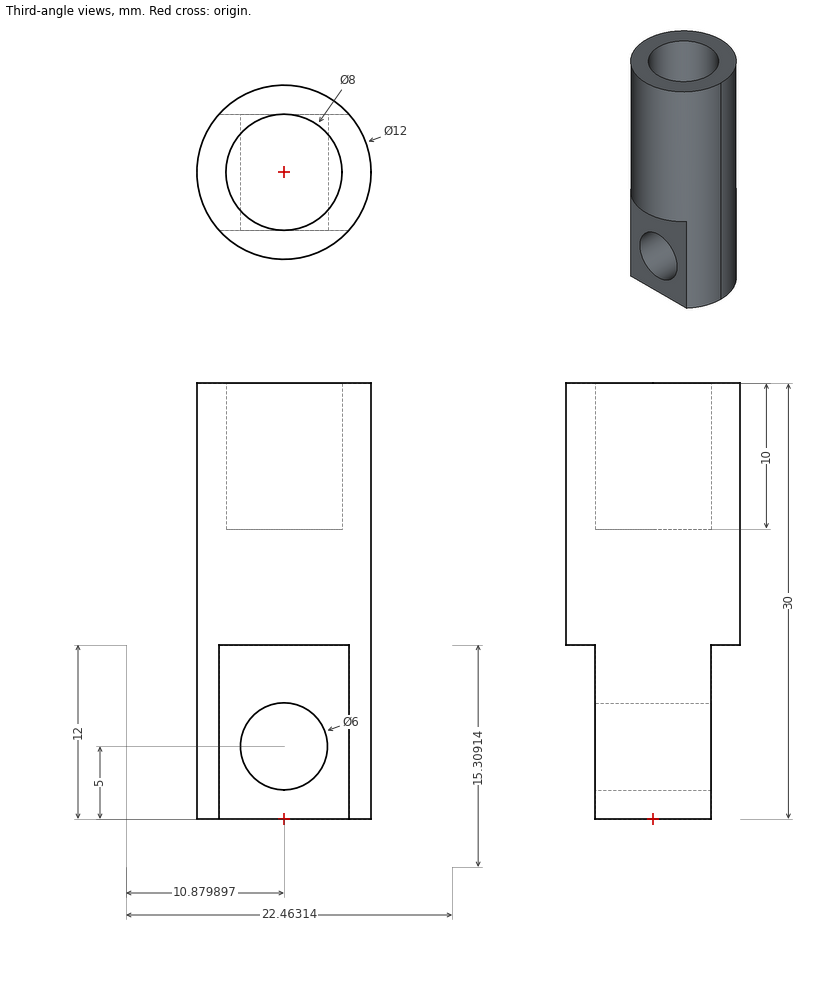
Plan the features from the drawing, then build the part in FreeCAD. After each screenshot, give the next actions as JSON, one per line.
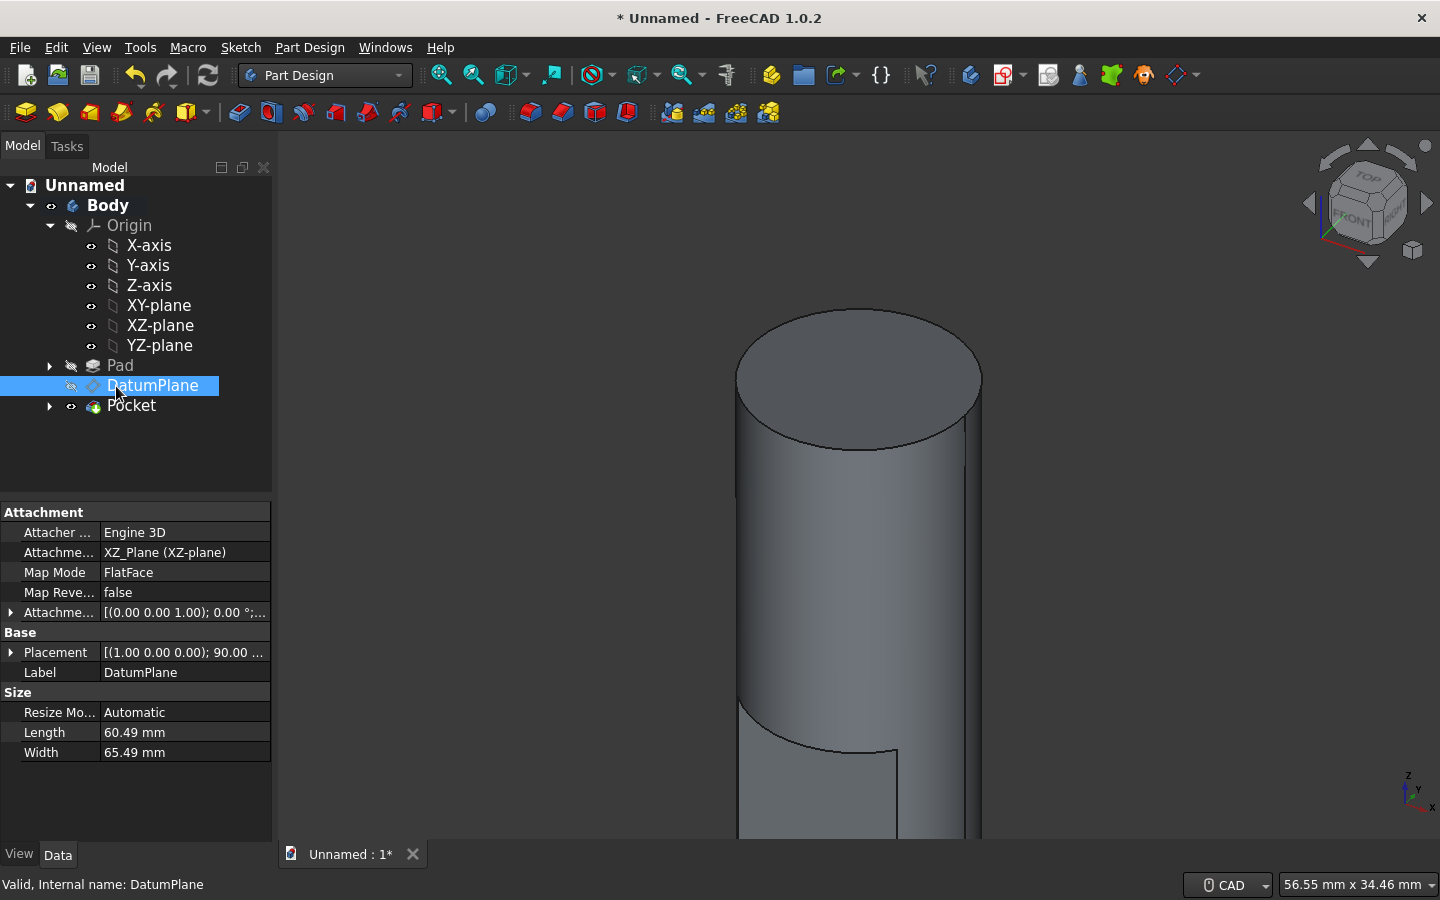
{"action": "left_click", "coordinate": [442, 76]}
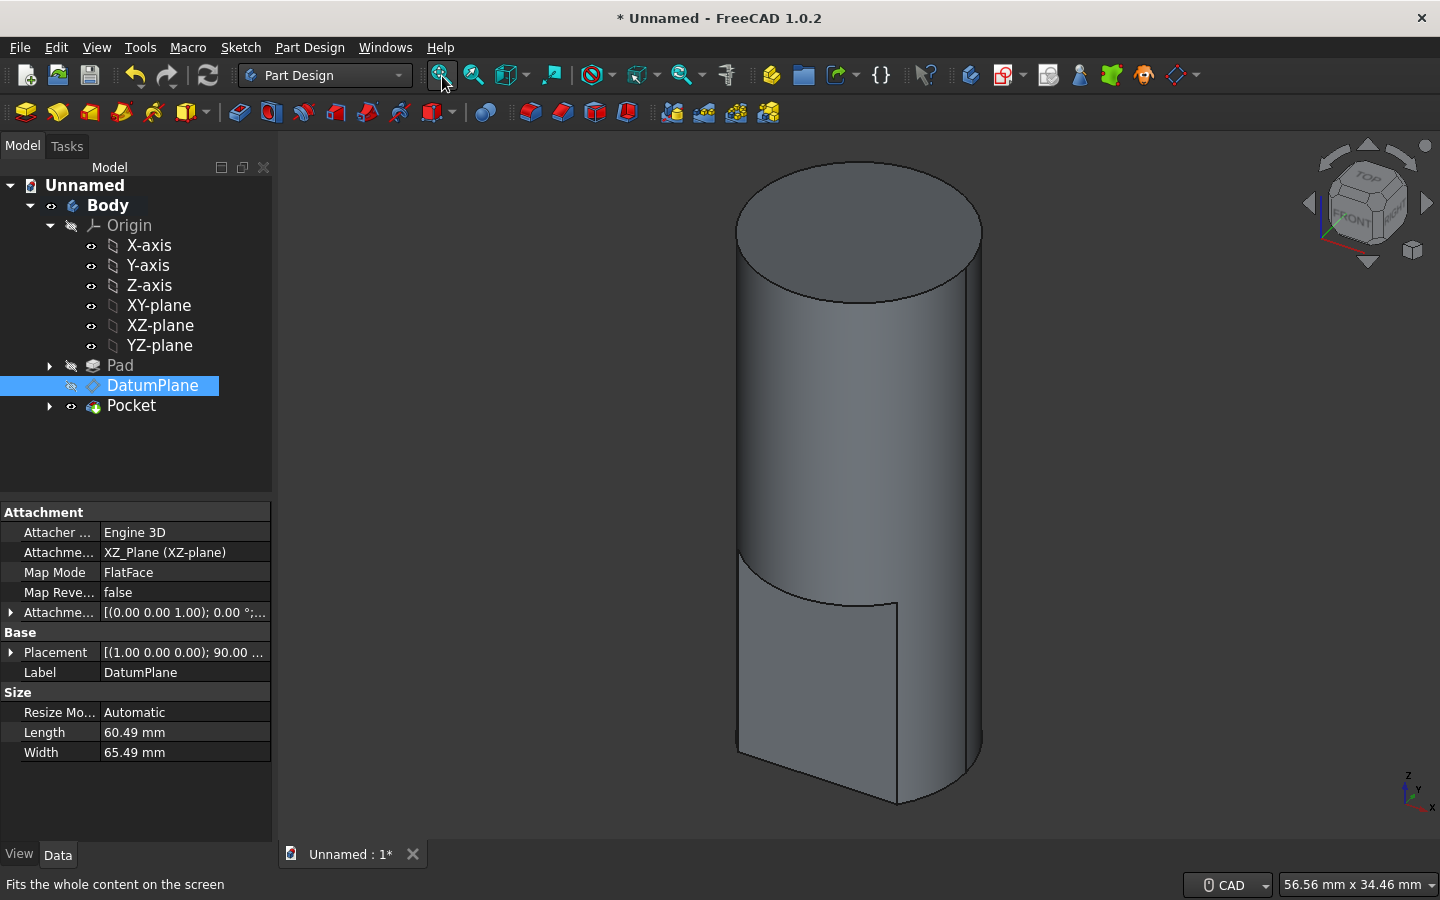
{"action": "left_click", "coordinate": [116, 406]}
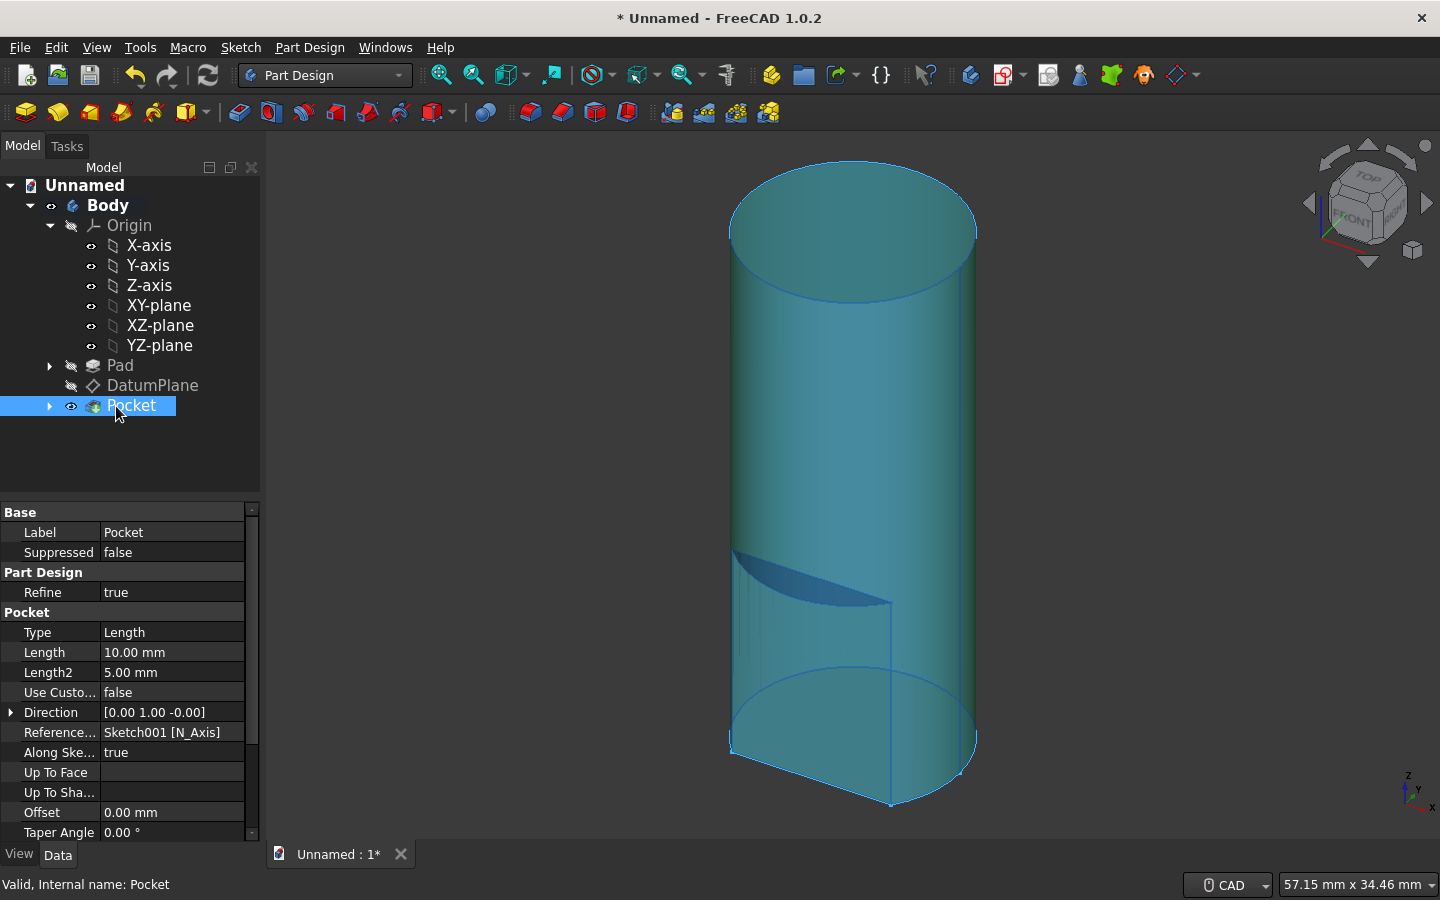
{"action": "left_click", "coordinate": [672, 112]}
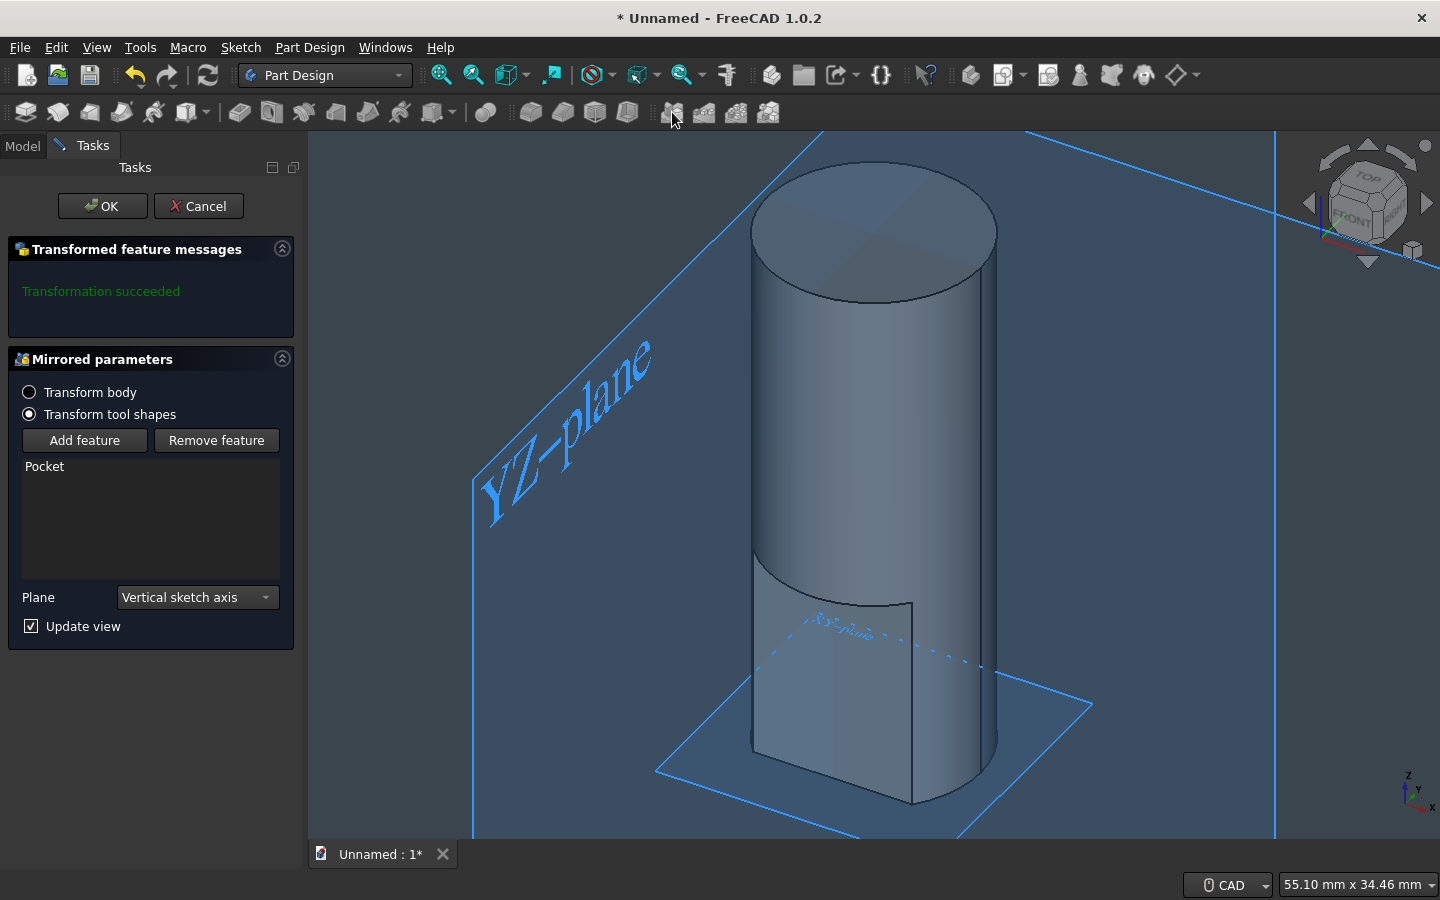
{"action": "left_click", "coordinate": [198, 598]}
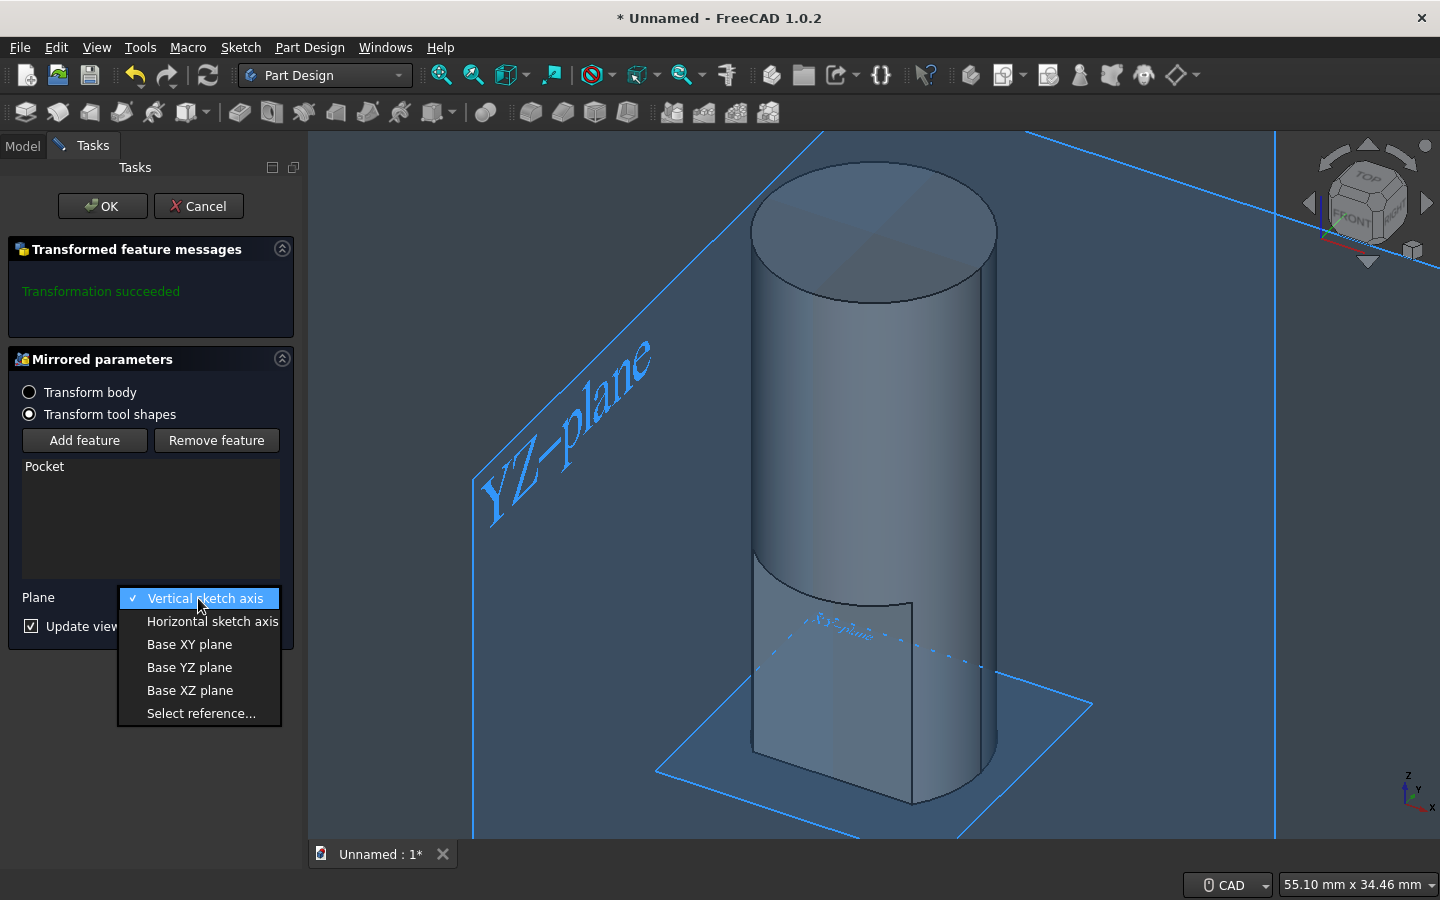
{"action": "left_click", "coordinate": [198, 690]}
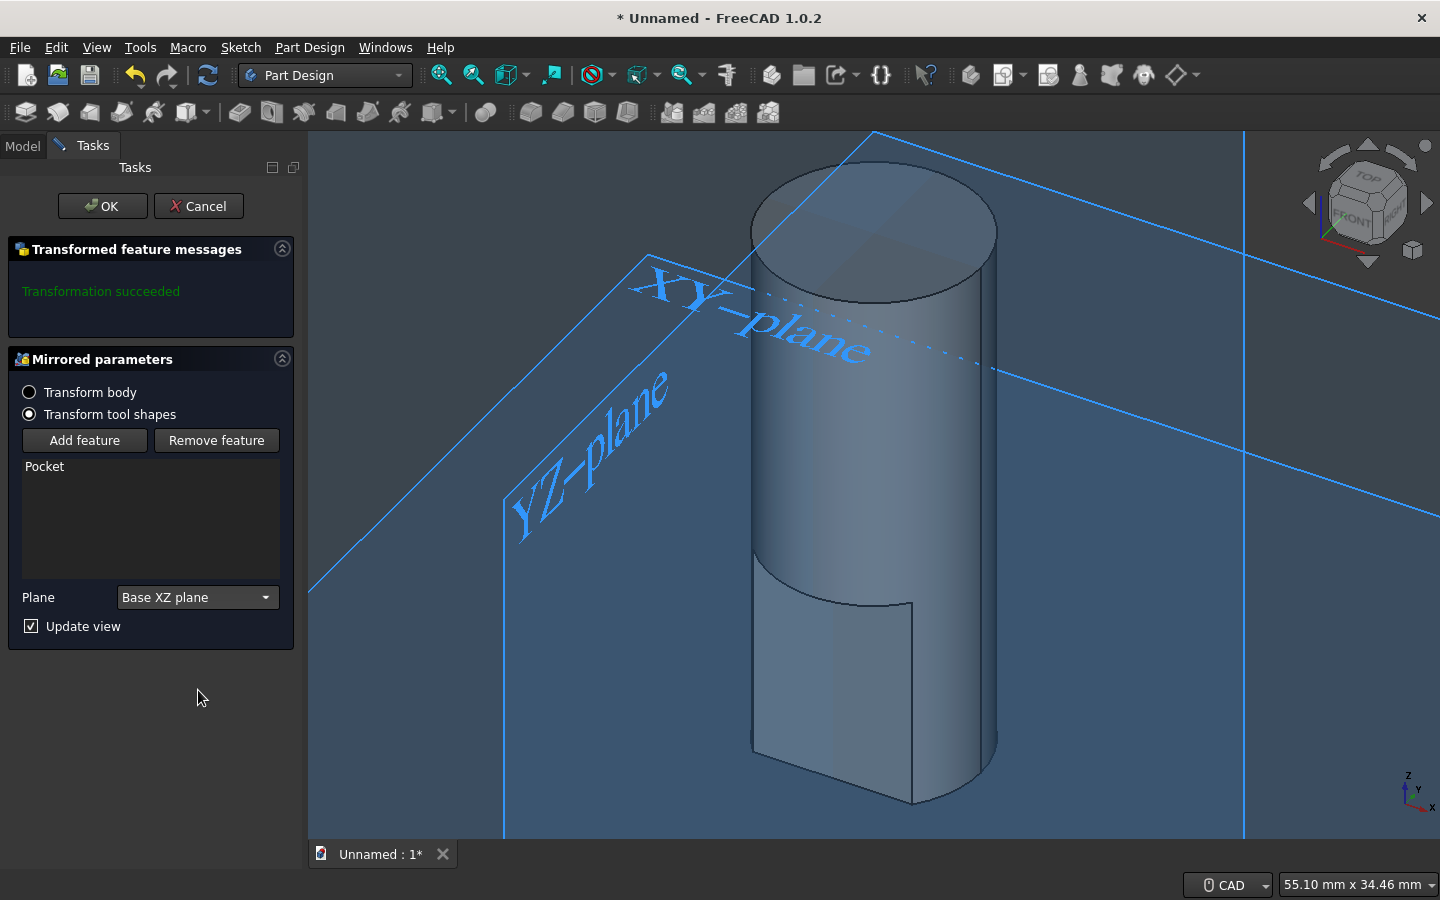
{"action": "left_click", "coordinate": [103, 206]}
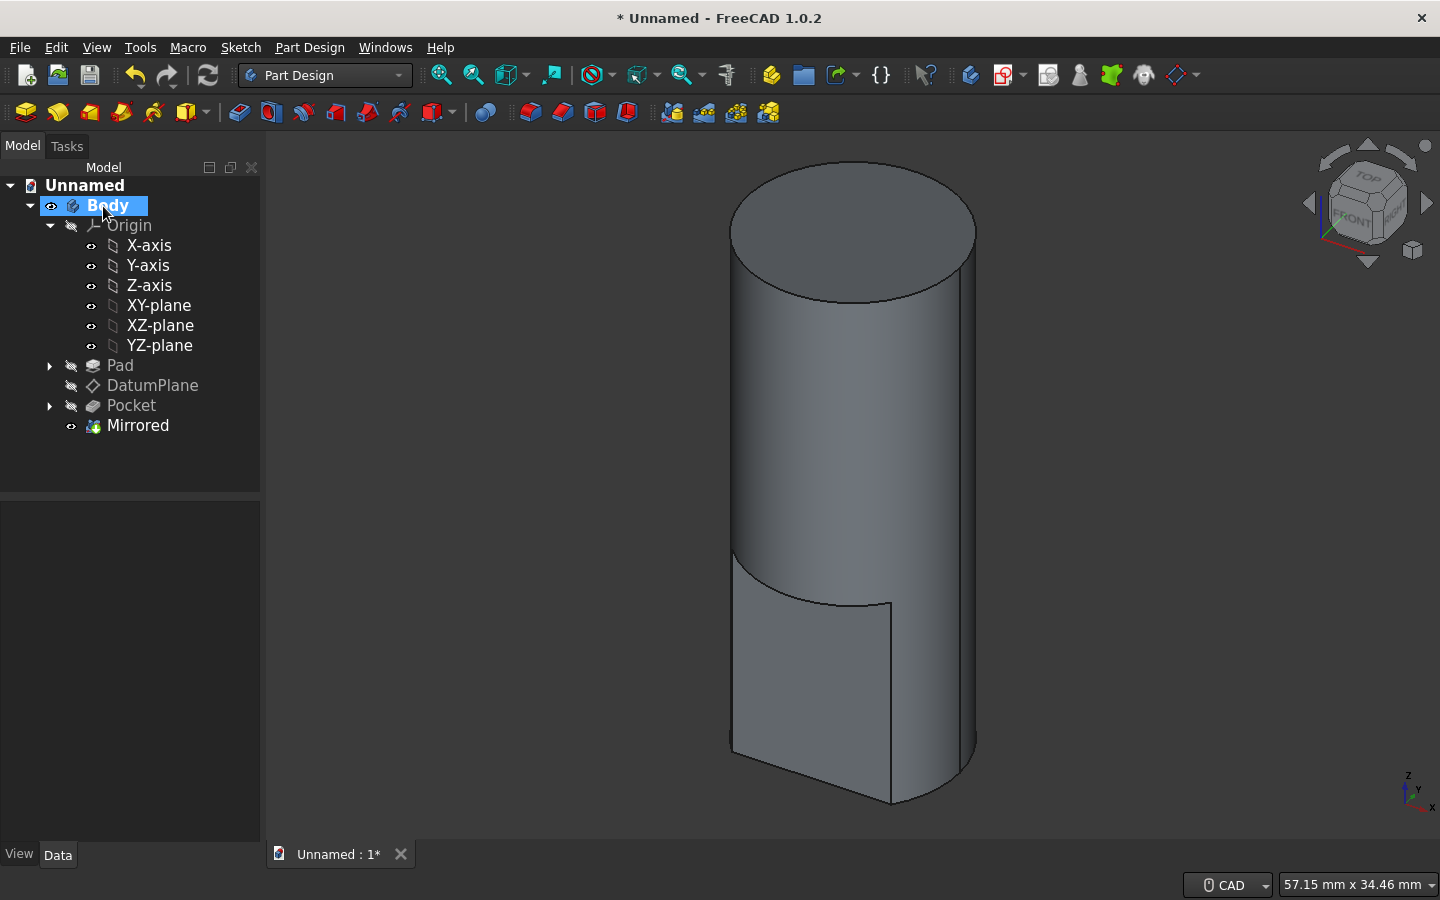
{"action": "left_click", "coordinate": [812, 676]}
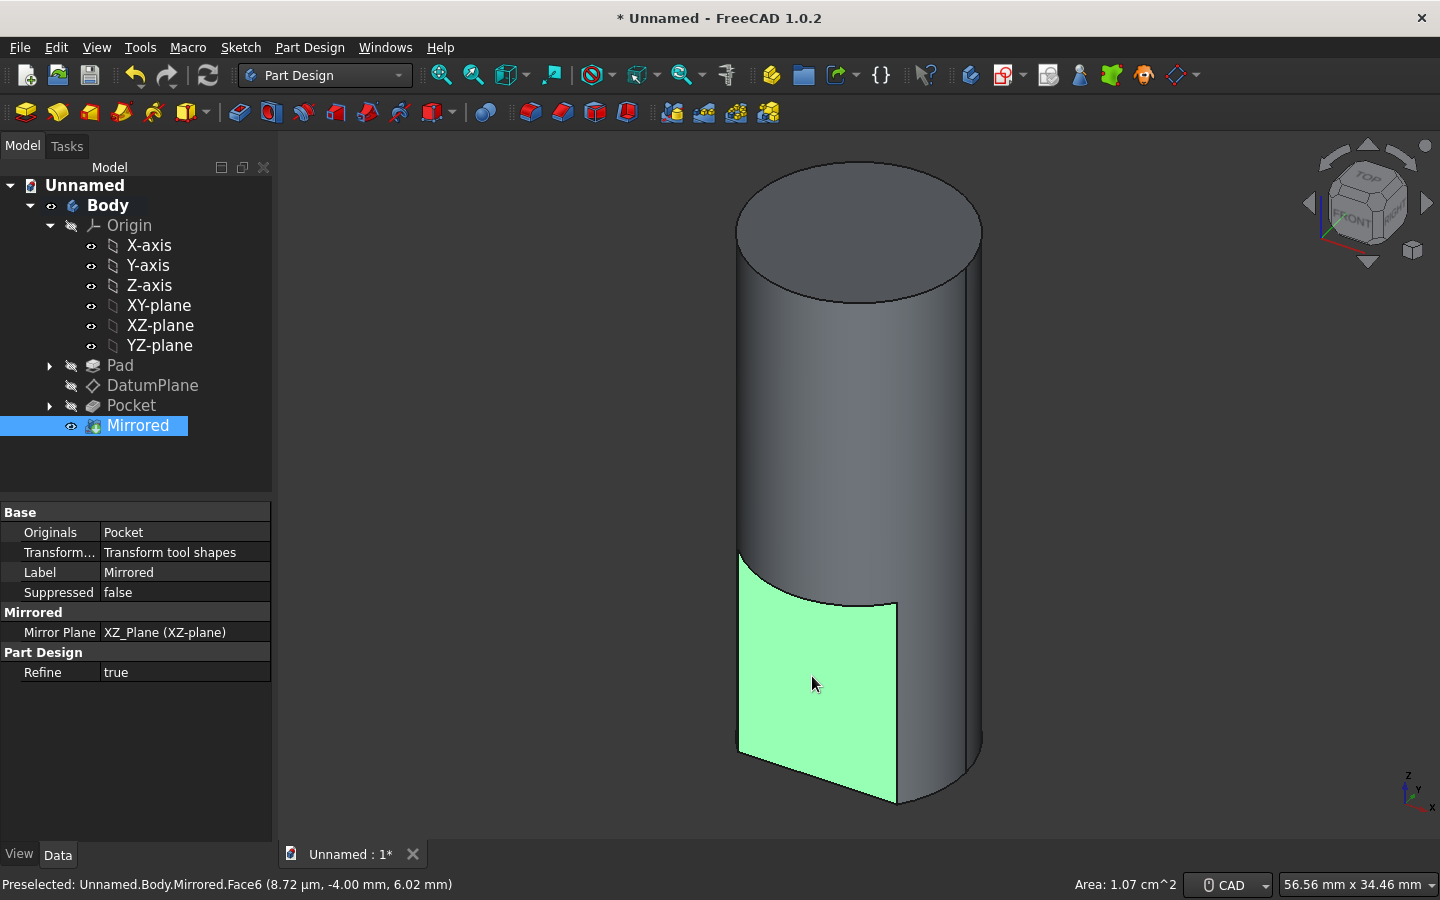
{"action": "left_click", "coordinate": [1004, 76]}